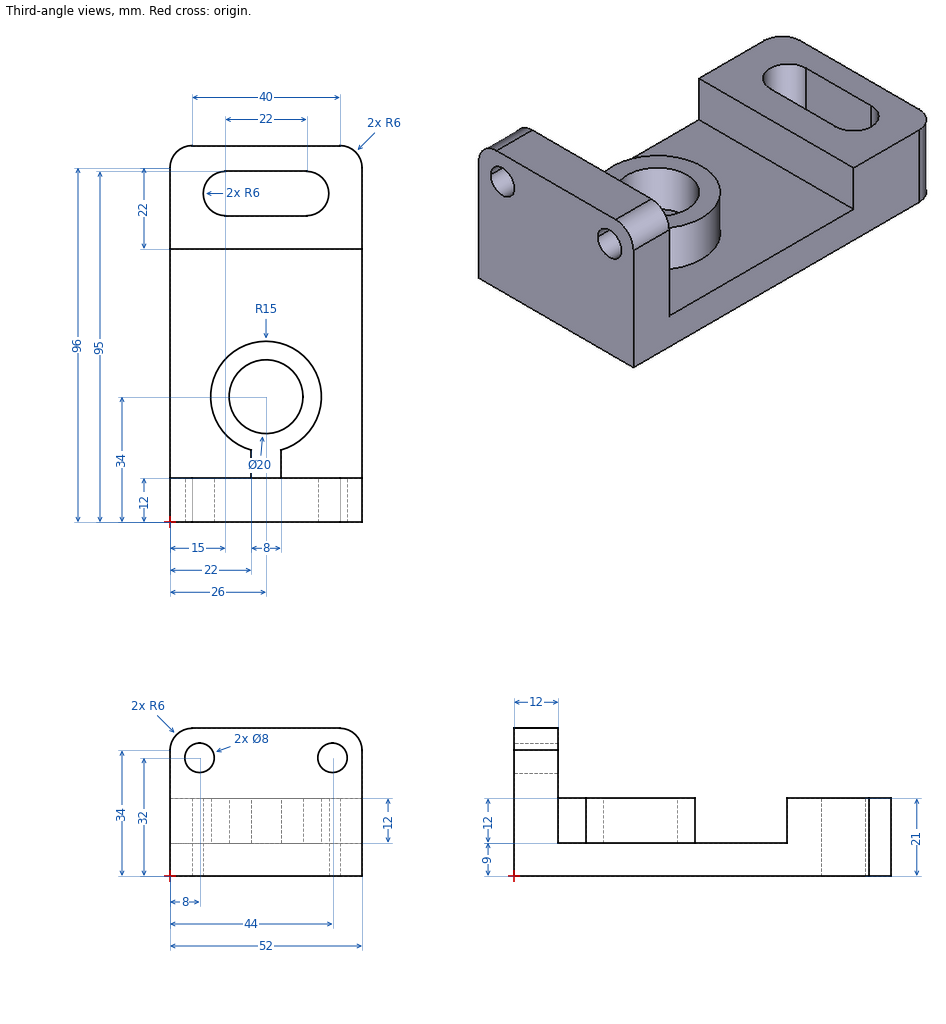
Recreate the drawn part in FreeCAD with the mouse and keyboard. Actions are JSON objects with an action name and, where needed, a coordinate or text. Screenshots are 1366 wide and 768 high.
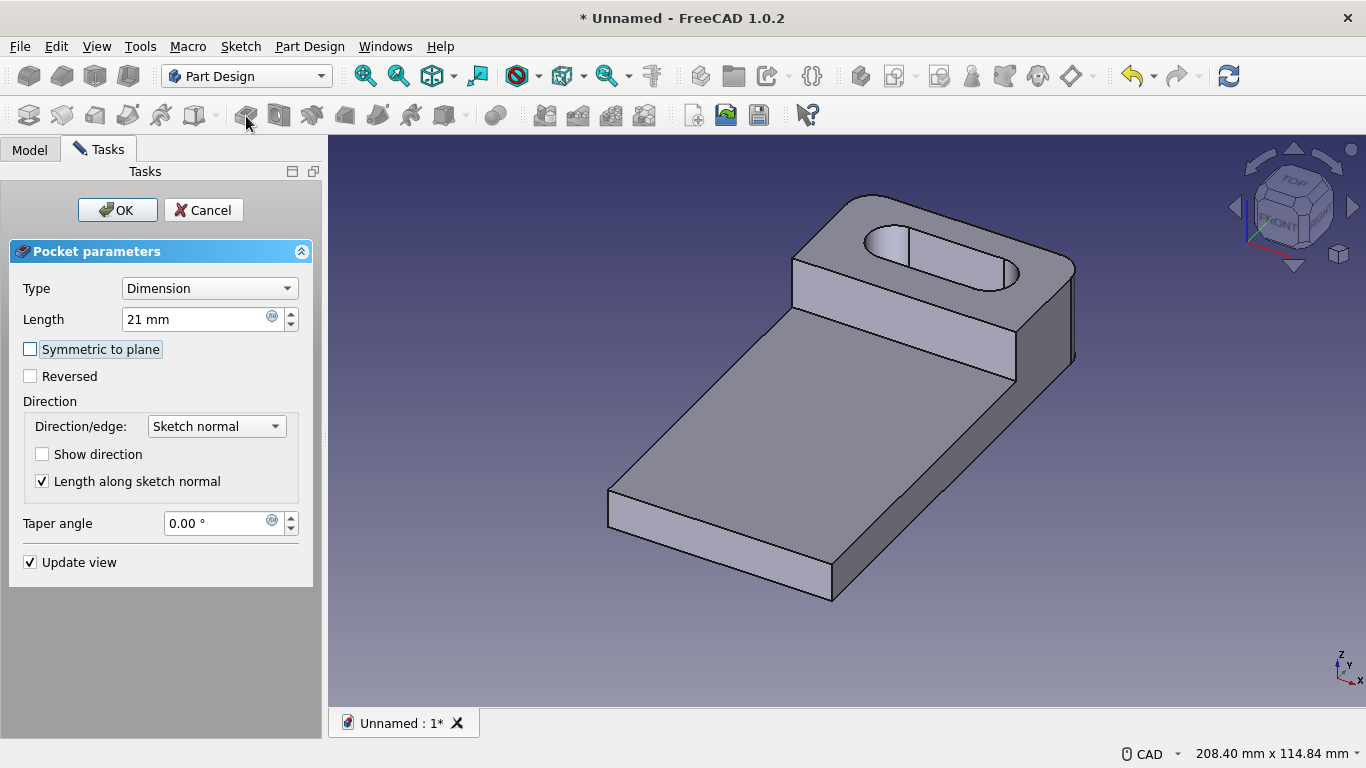
{"action": "left_click", "coordinate": [118, 210]}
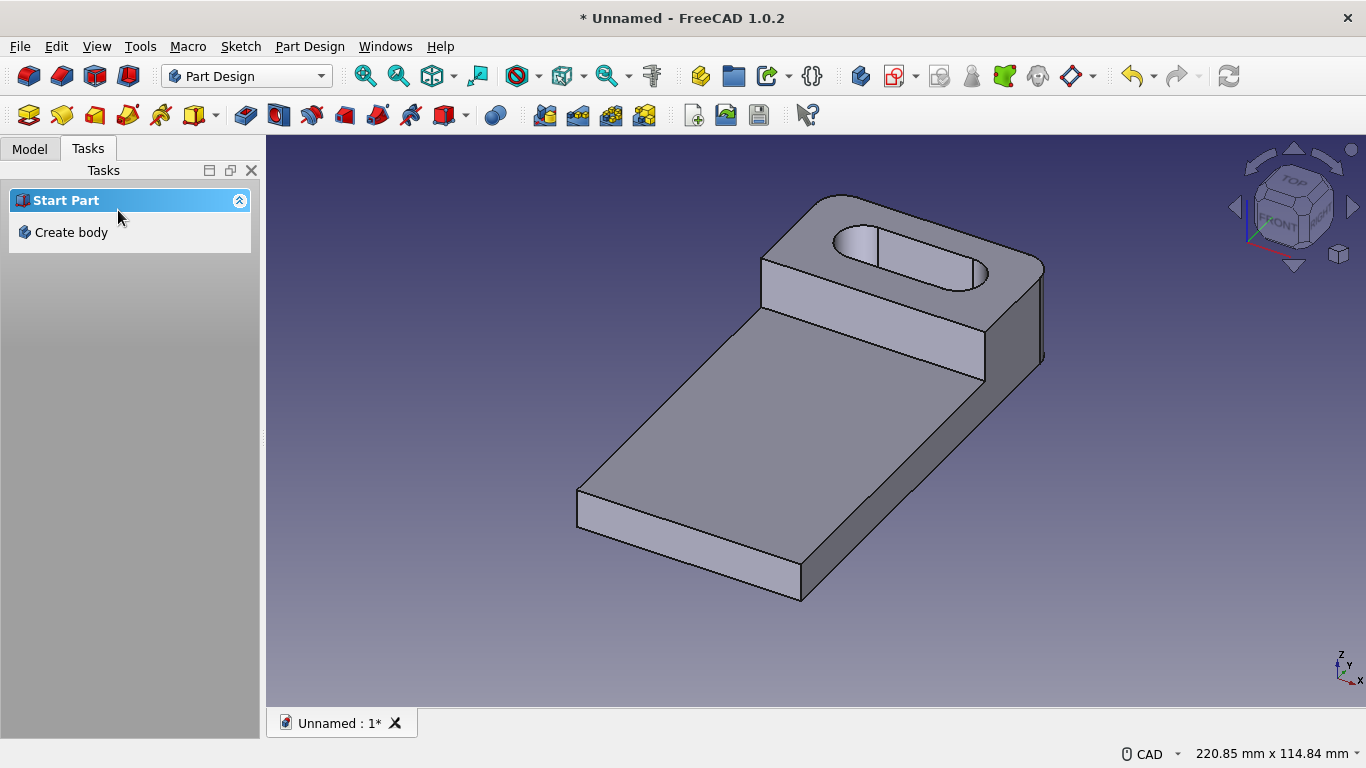
{"action": "left_click", "coordinate": [894, 76]}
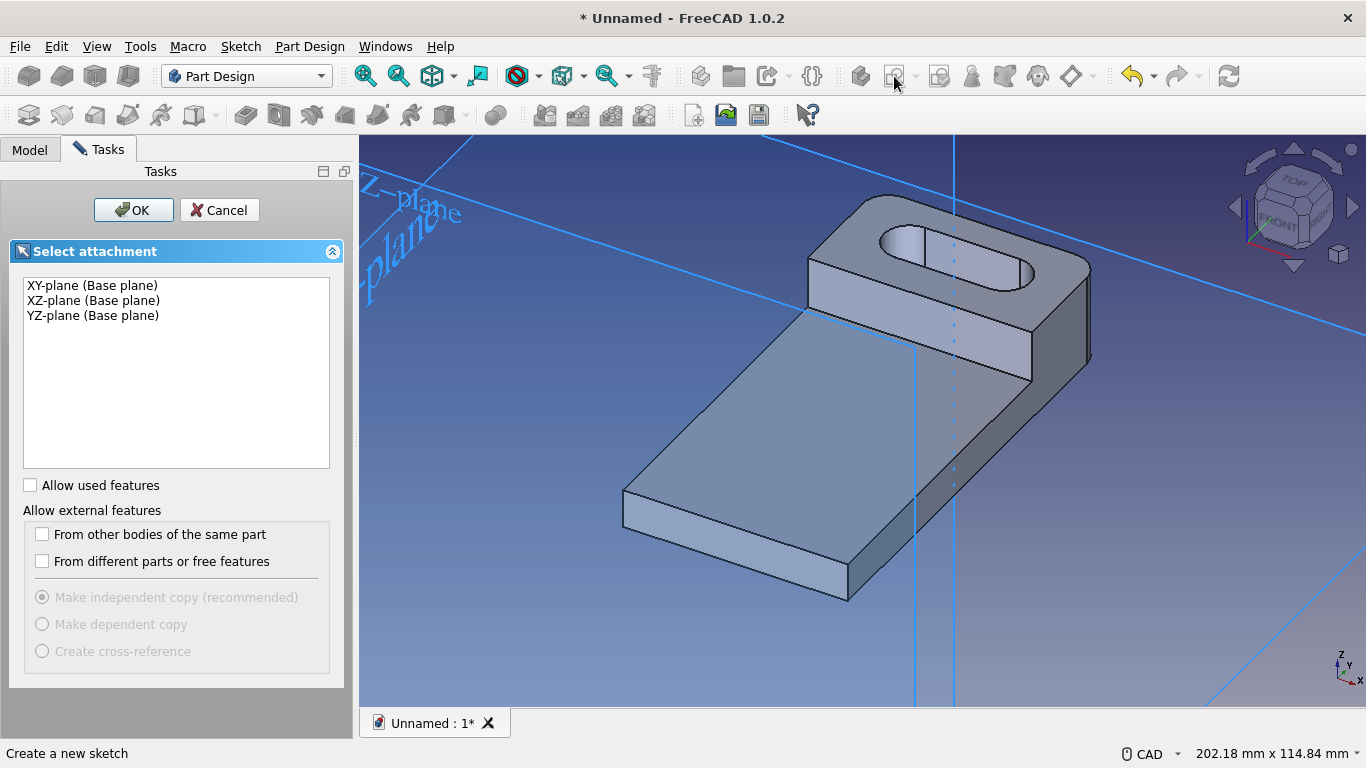
{"action": "left_click", "coordinate": [84, 300]}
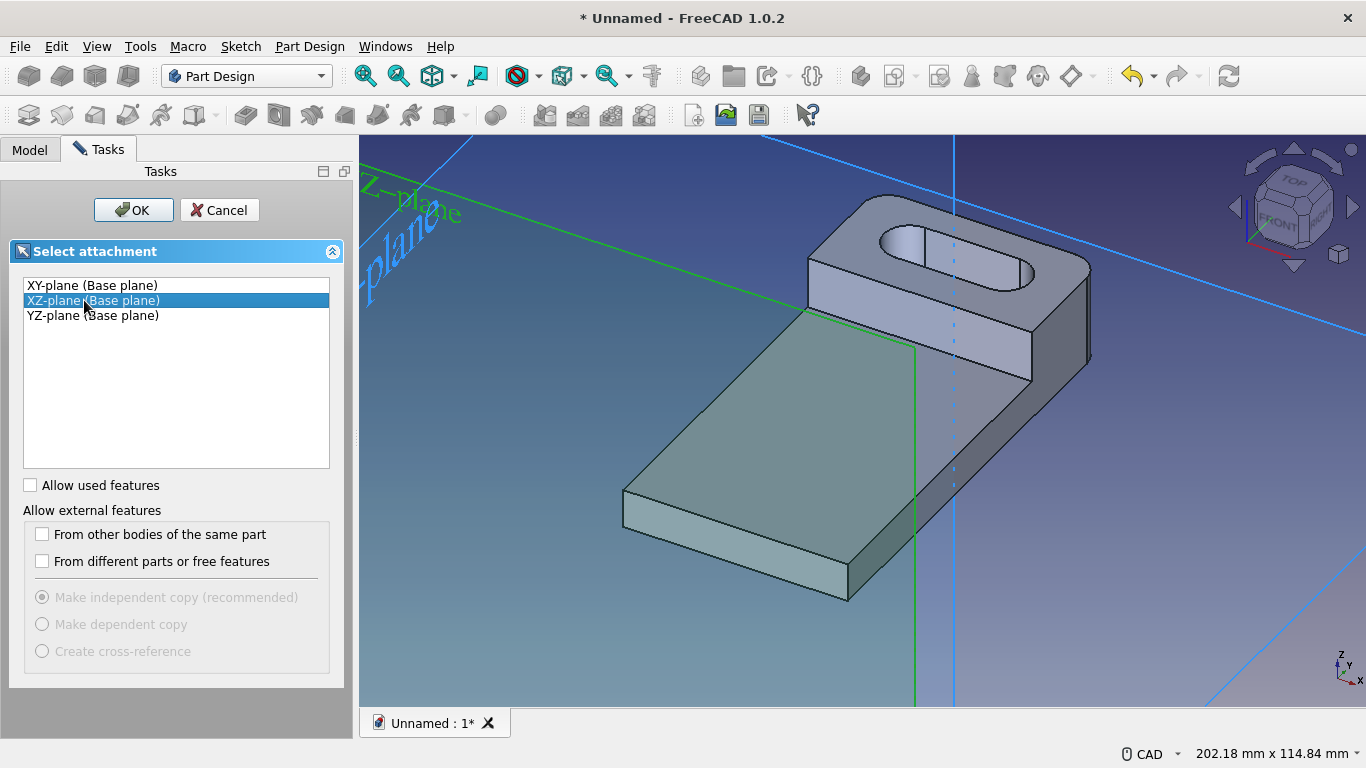
{"action": "left_click", "coordinate": [134, 210]}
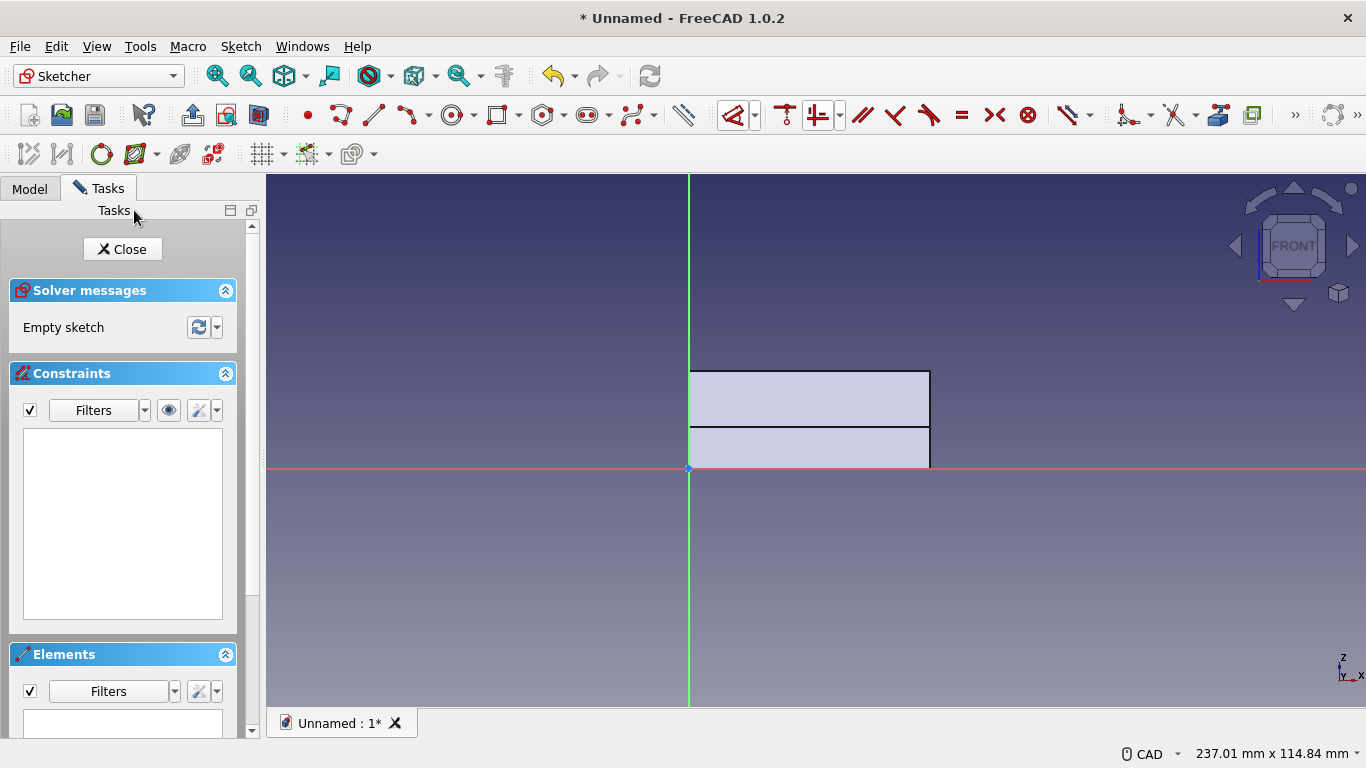
{"action": "scroll", "coordinate": [885, 297], "scroll_direction": "up", "scroll_amount": 3}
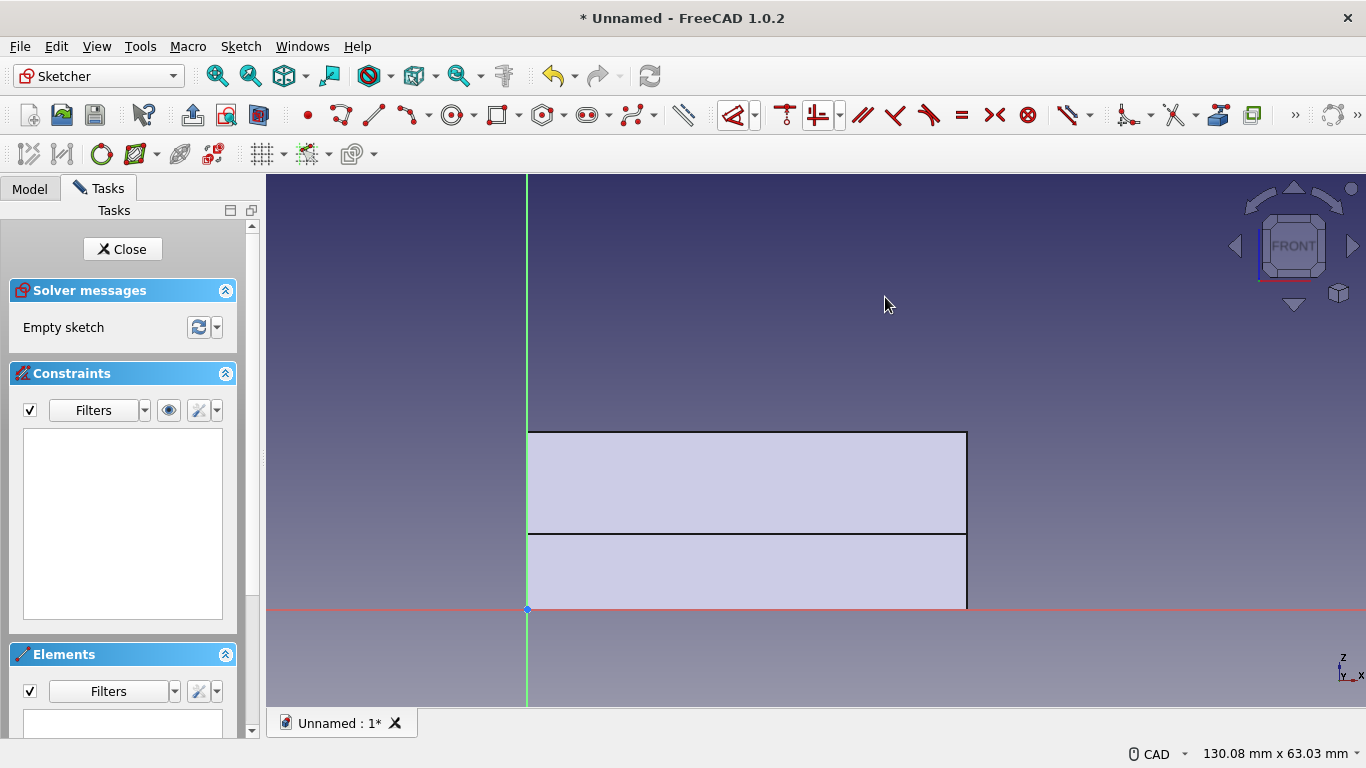
{"action": "left_click", "coordinate": [341, 116]}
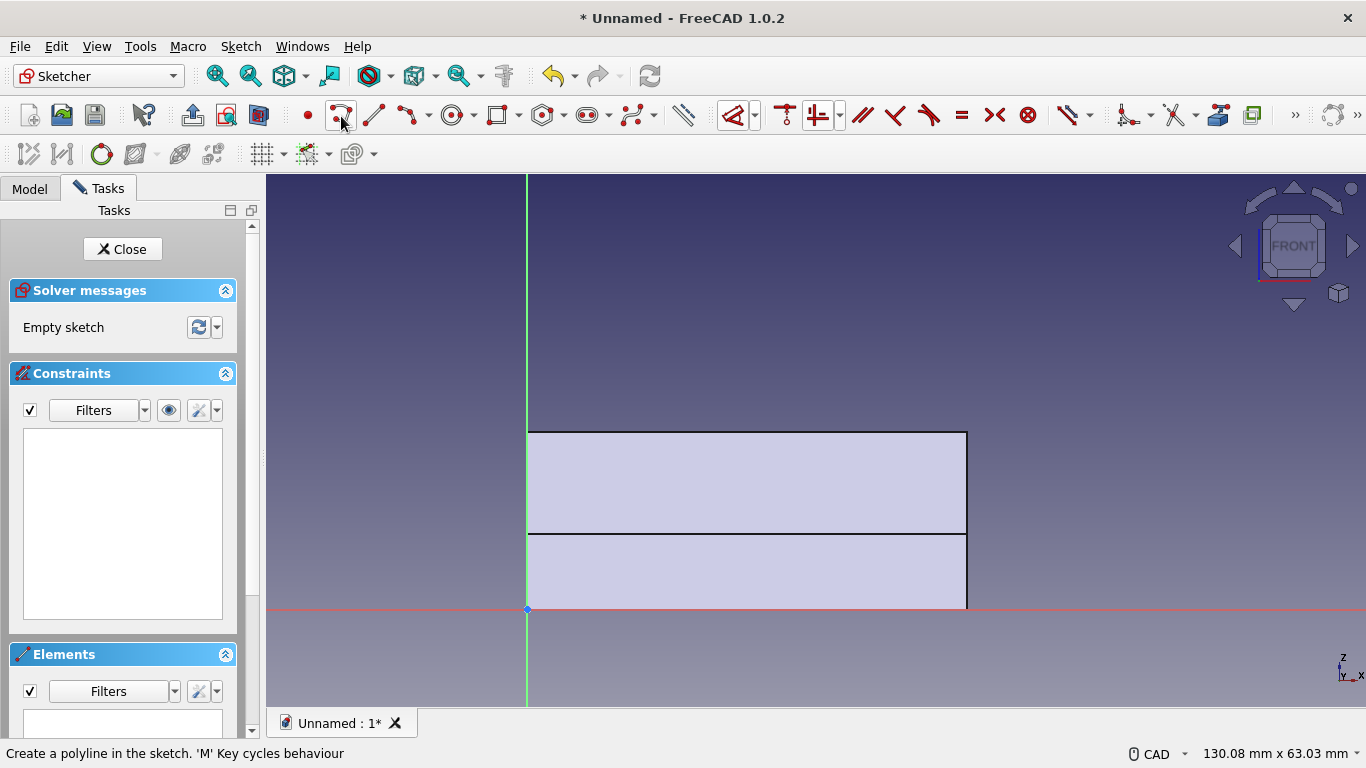
{"action": "left_click", "coordinate": [527, 322]}
{"action": "left_click", "coordinate": [527, 610]}
{"action": "left_click", "coordinate": [967, 601]}
{"action": "left_click", "coordinate": [967, 322]}
{"action": "right_click", "coordinate": [967, 322]}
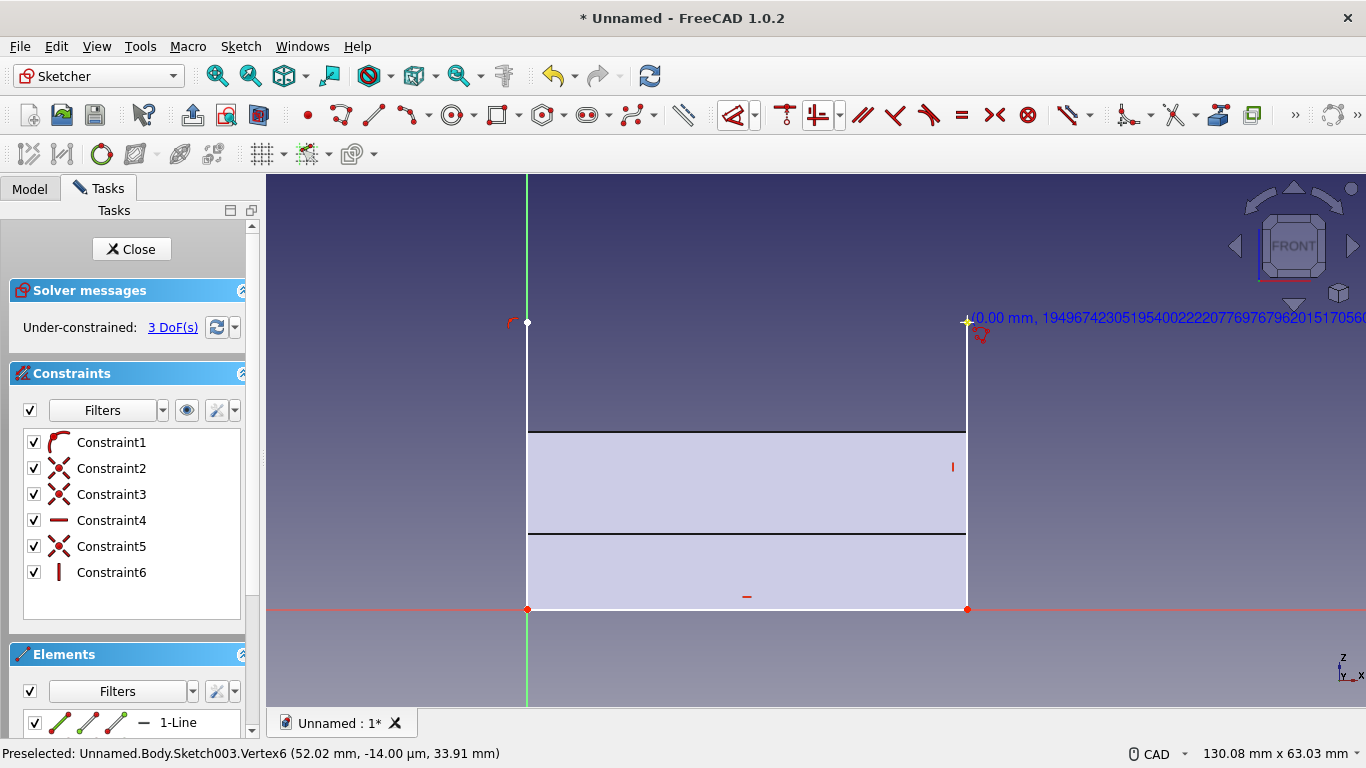
{"action": "left_click", "coordinate": [374, 116]}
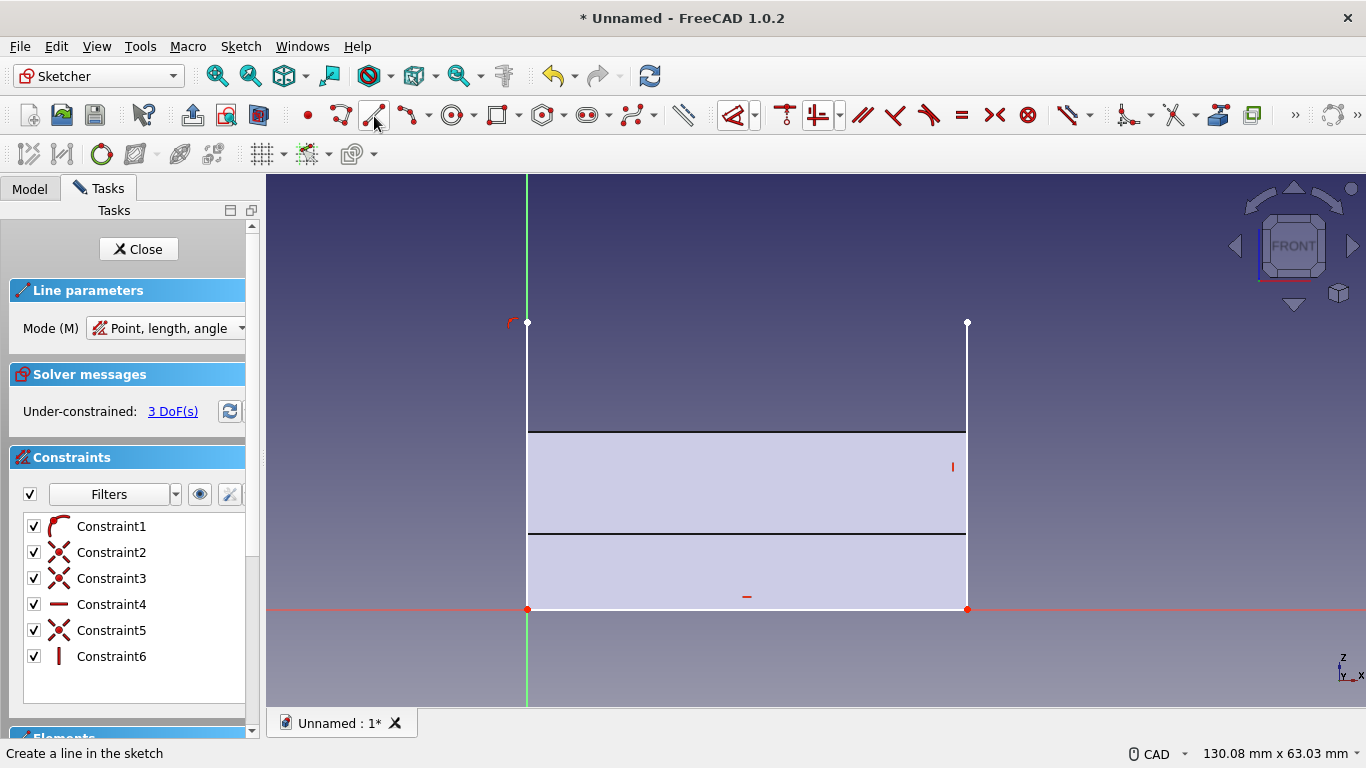
{"action": "left_click", "coordinate": [916, 271]}
{"action": "left_click", "coordinate": [578, 271]}